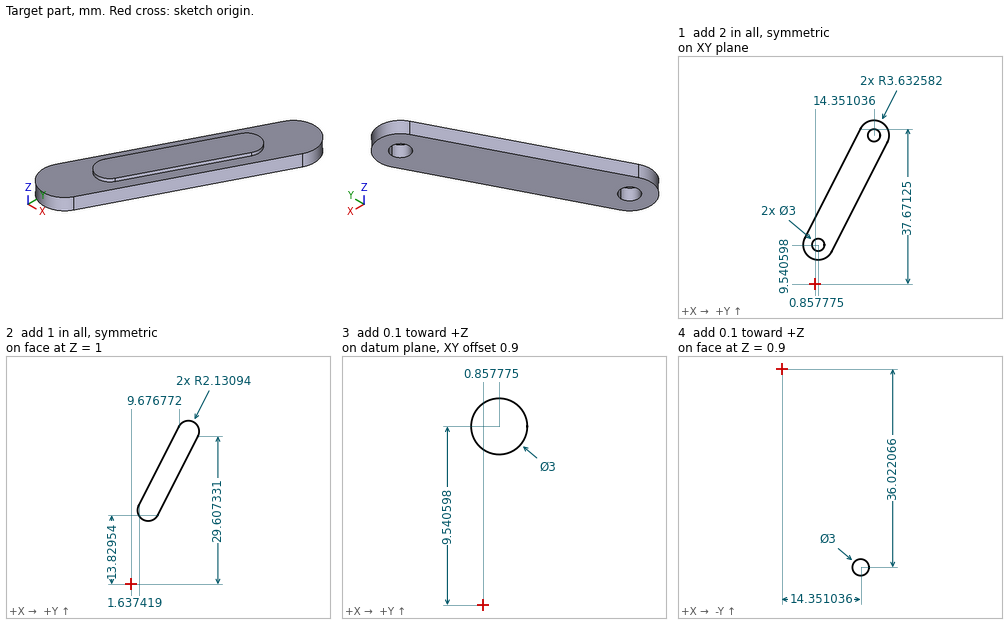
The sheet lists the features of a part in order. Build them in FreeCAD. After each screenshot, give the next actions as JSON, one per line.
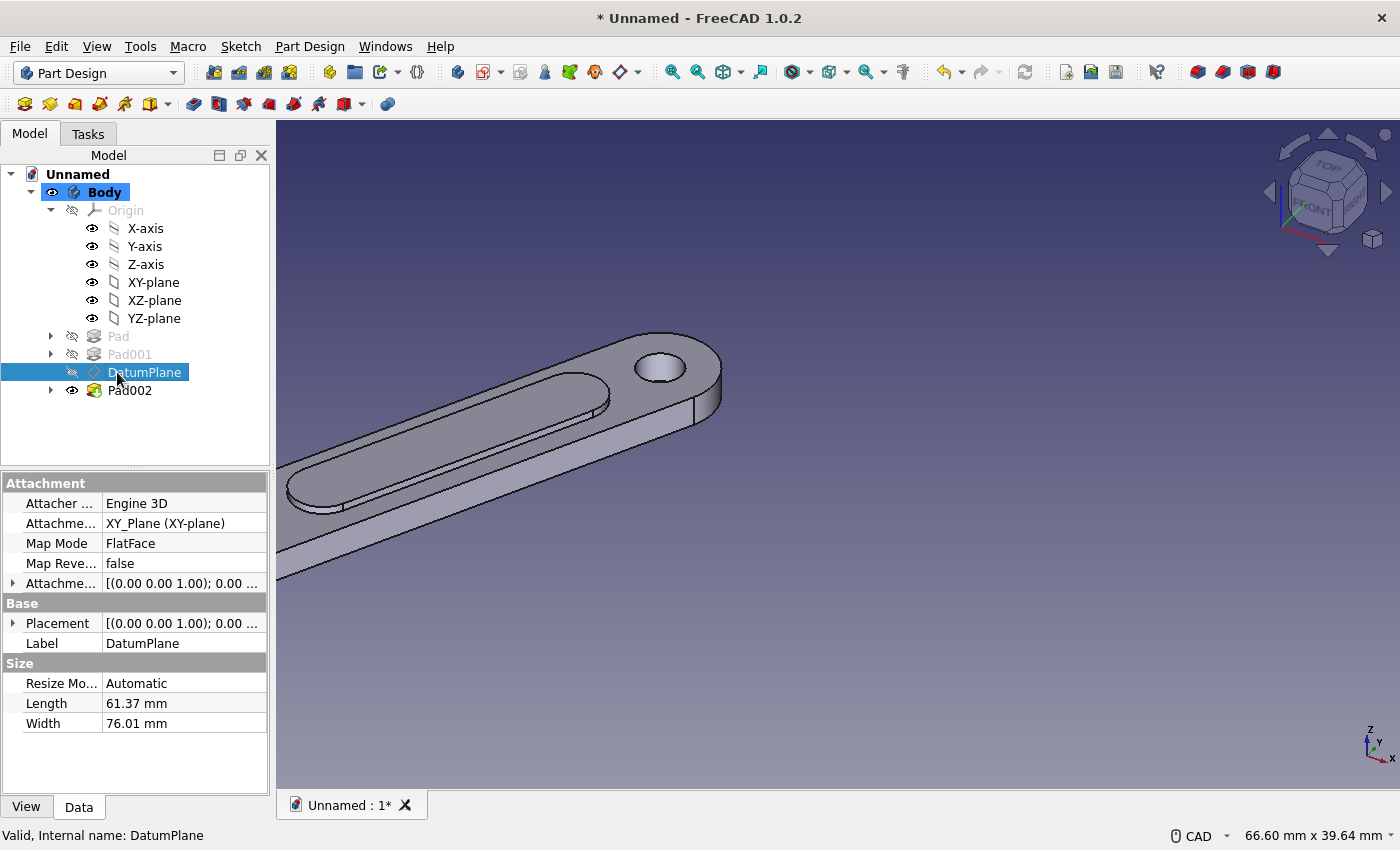
{"action": "key", "text": "v f"}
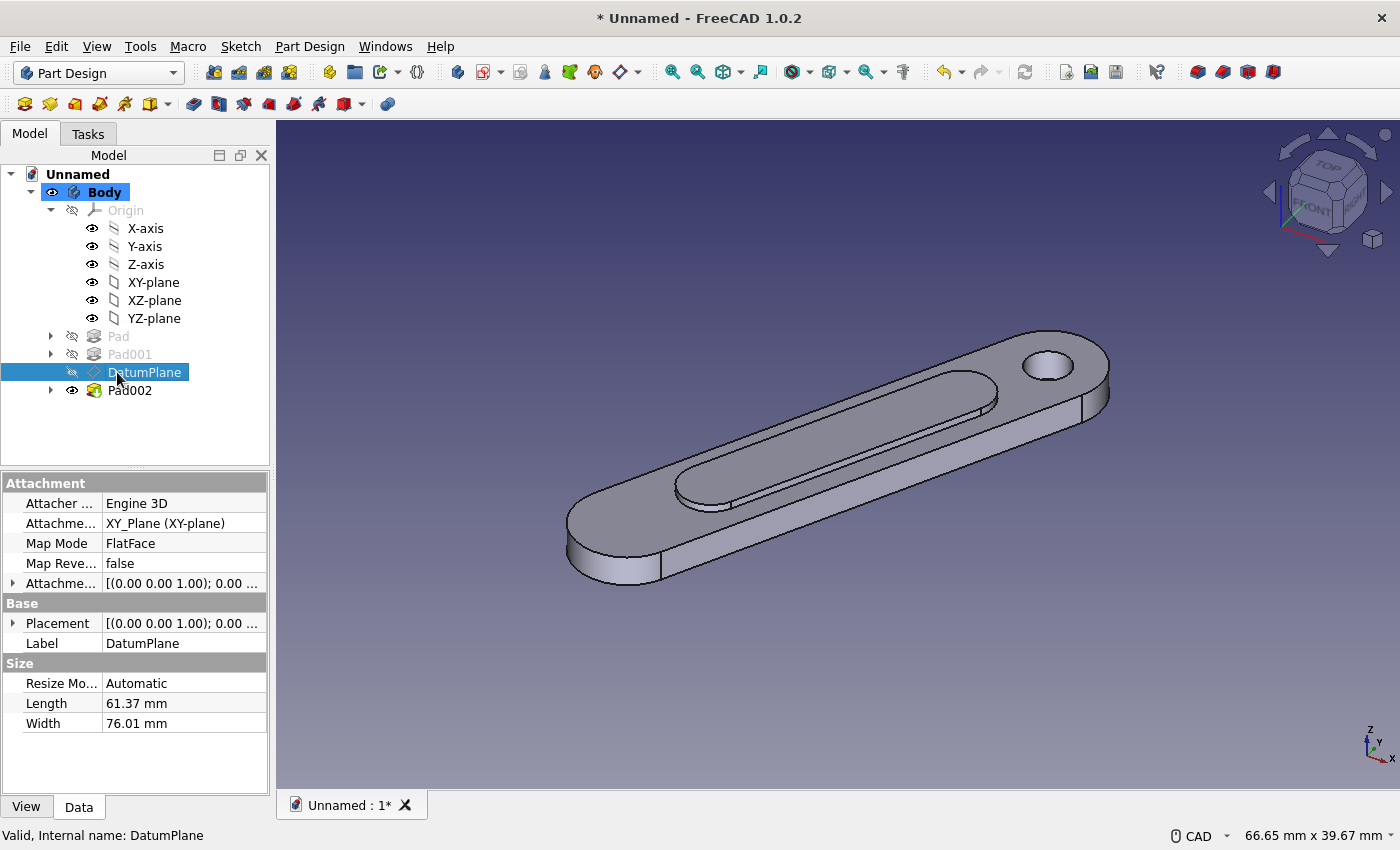
{"action": "key", "text": "5"}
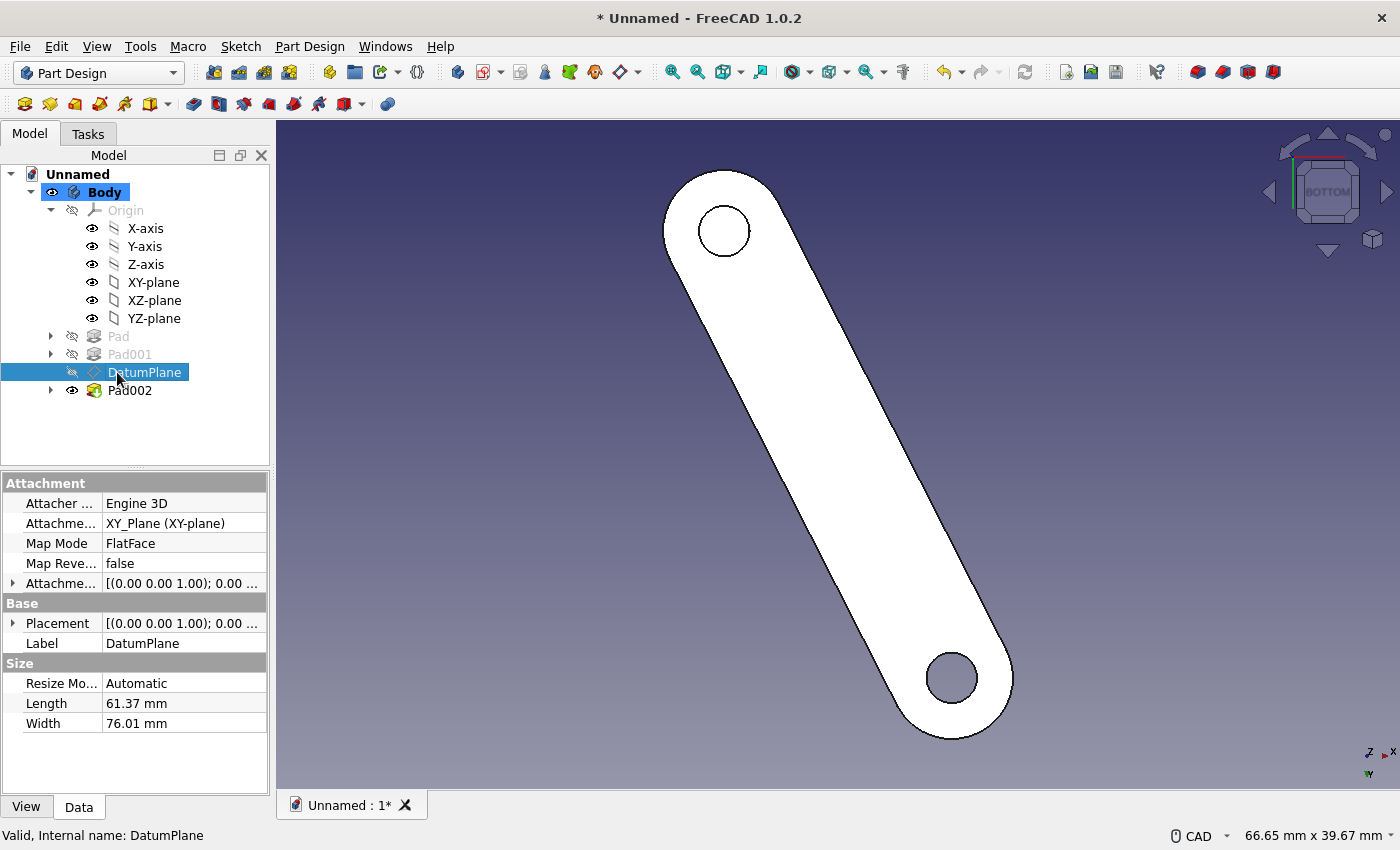
{"action": "left_click", "coordinate": [724, 230]}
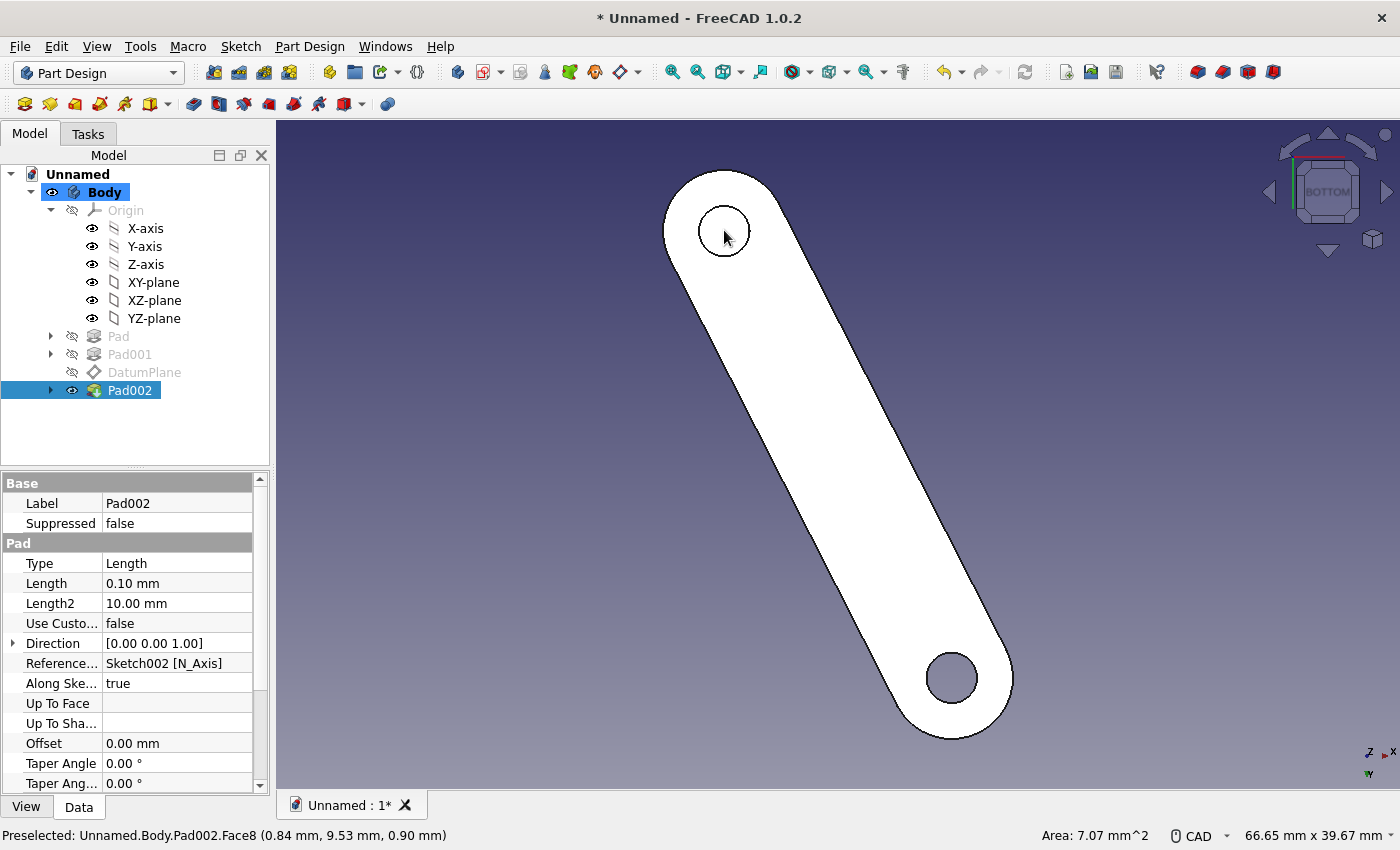
{"action": "left_click", "coordinate": [482, 72]}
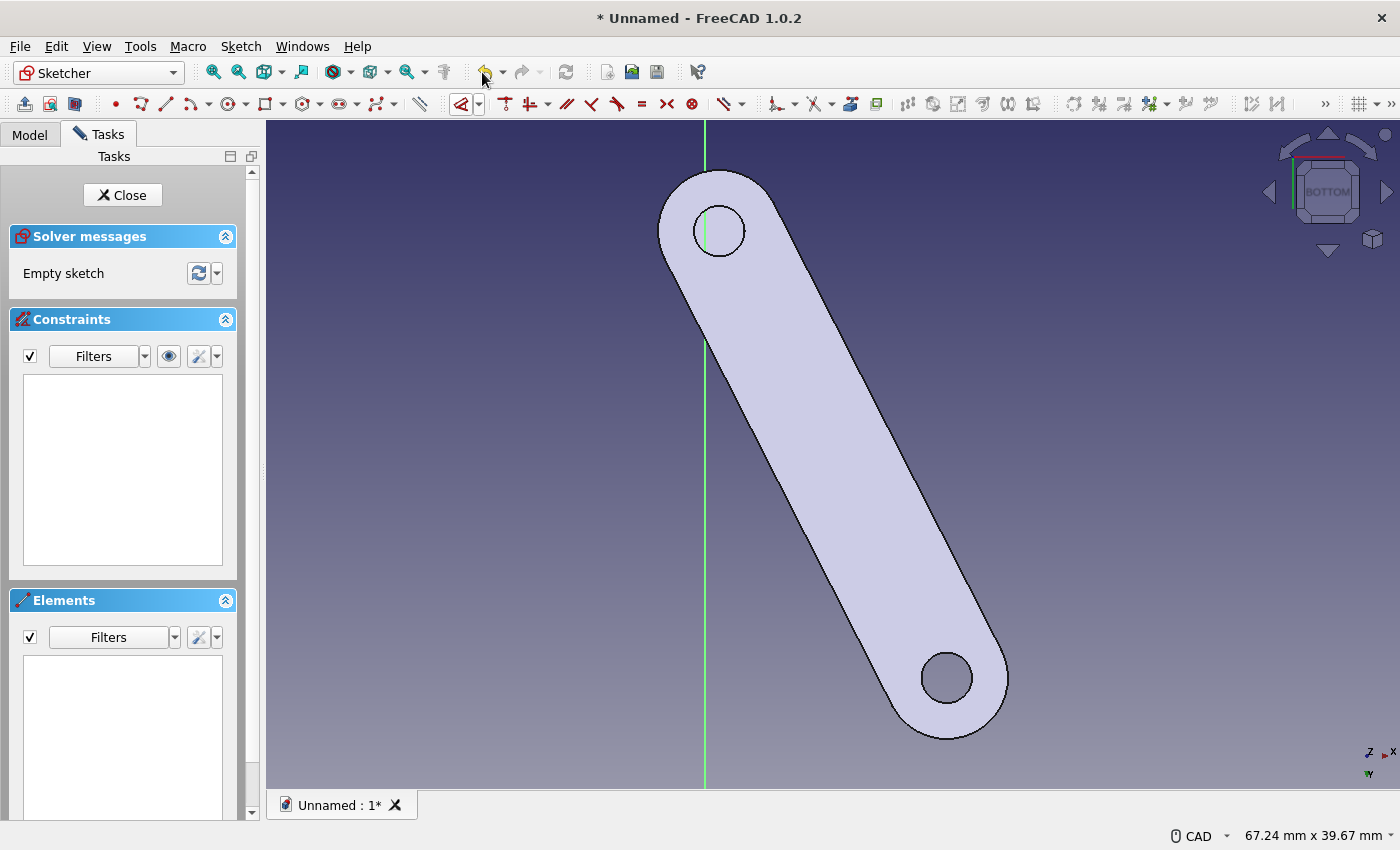
{"action": "scroll", "coordinate": [969, 706], "scroll_direction": "up", "scroll_amount": 11}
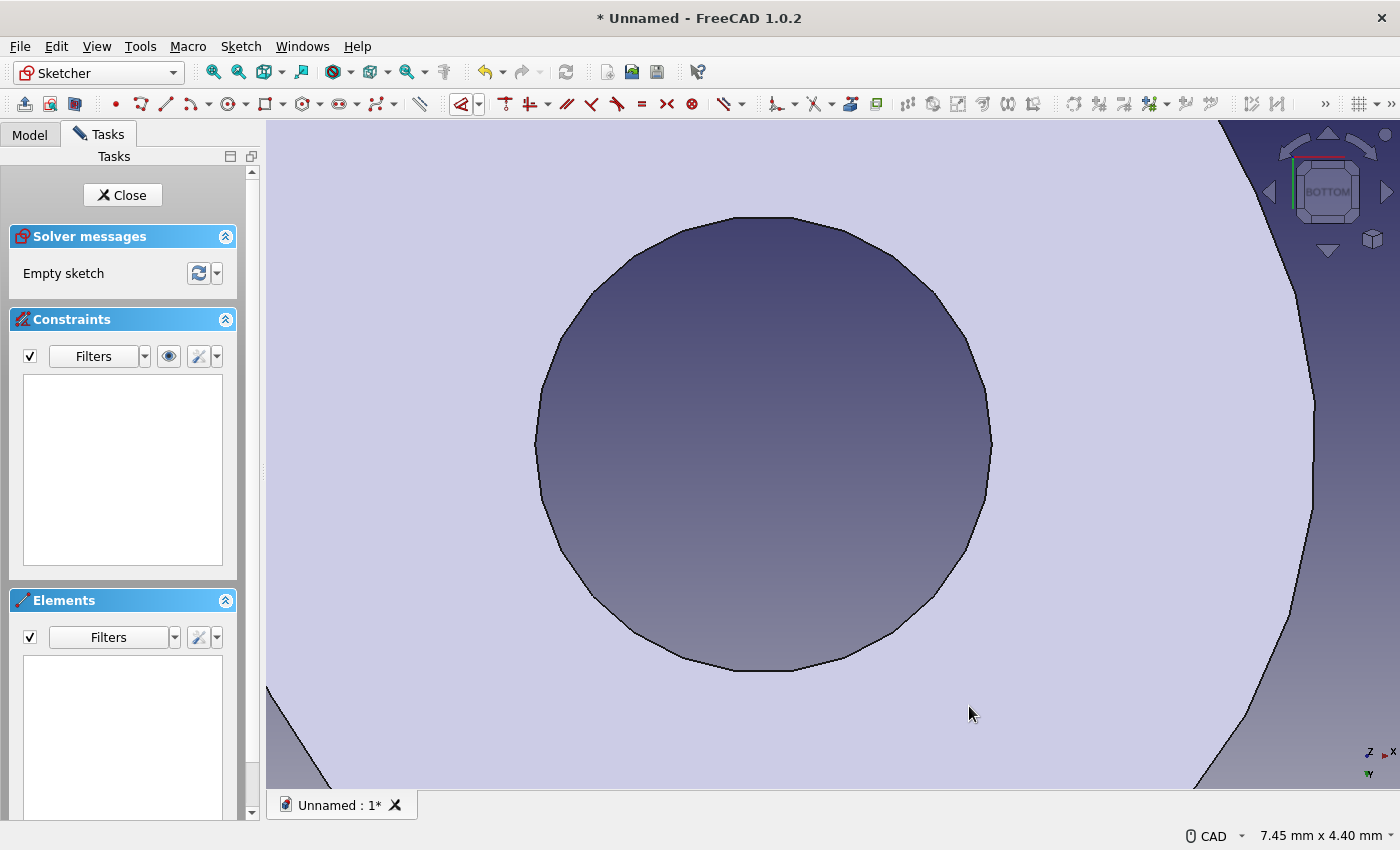
{"action": "key", "text": "g c"}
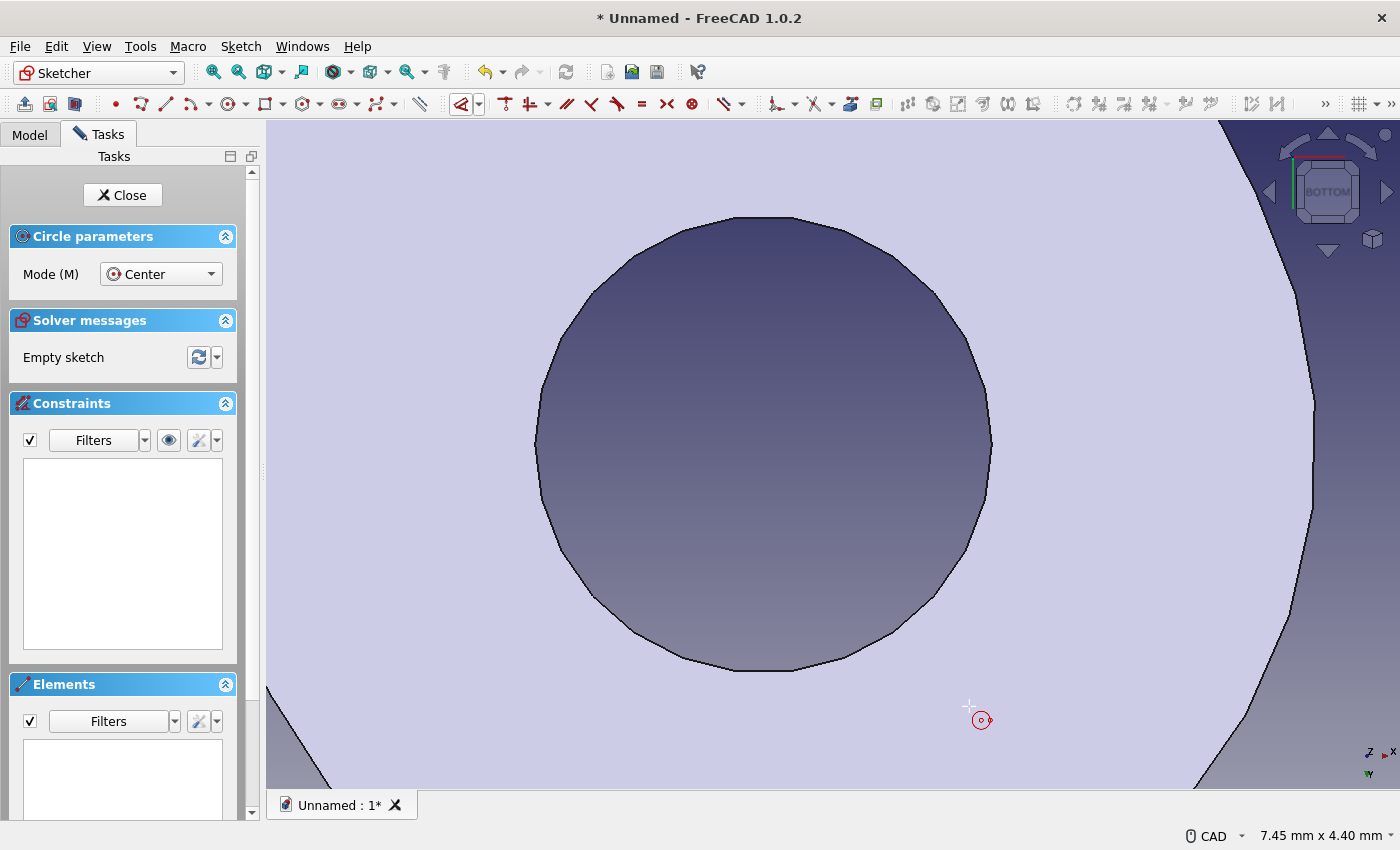
{"action": "left_click", "coordinate": [763, 444]}
{"action": "left_click", "coordinate": [925, 283]}
{"action": "key", "text": "Escape"}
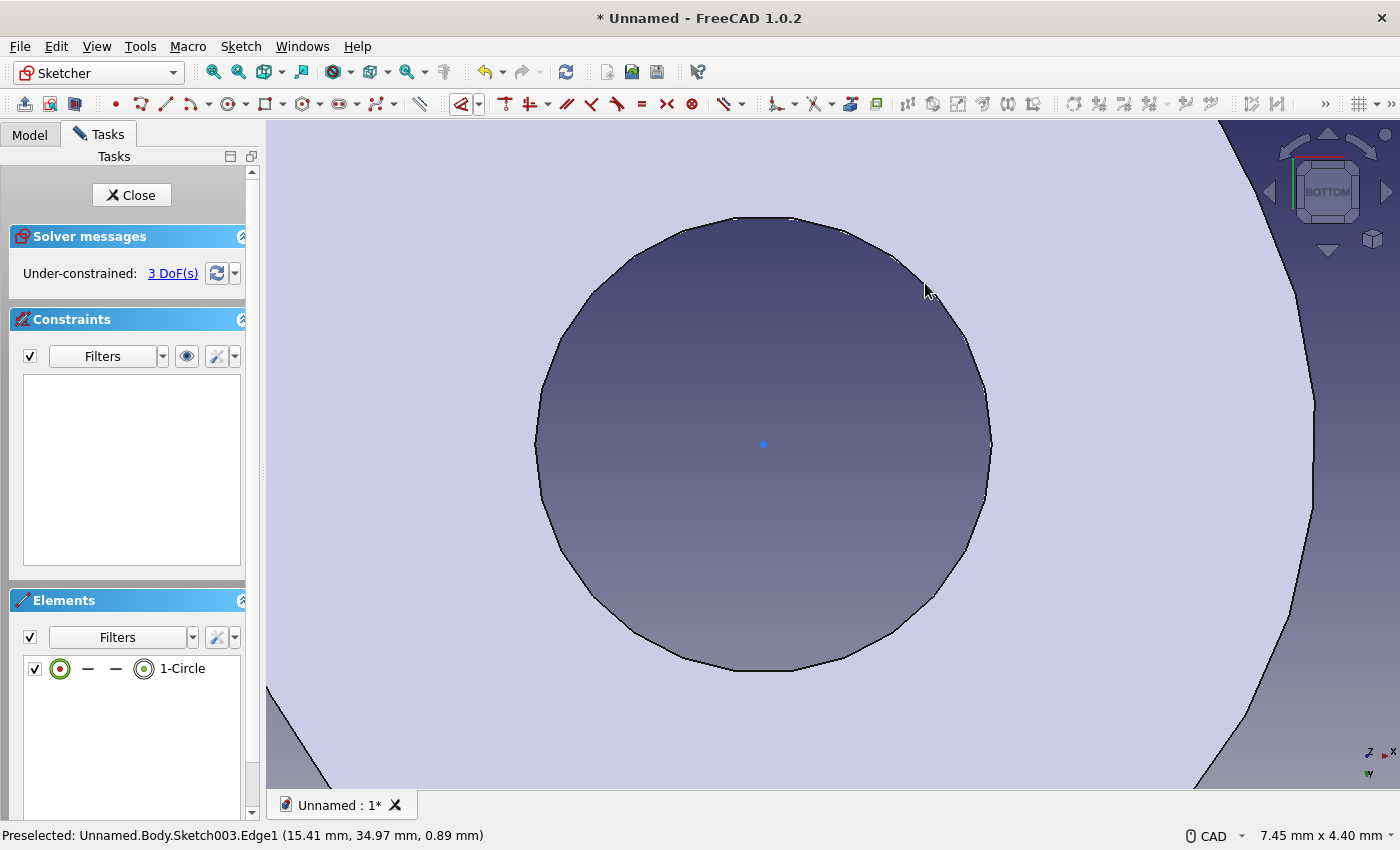
{"action": "left_click", "coordinate": [924, 283]}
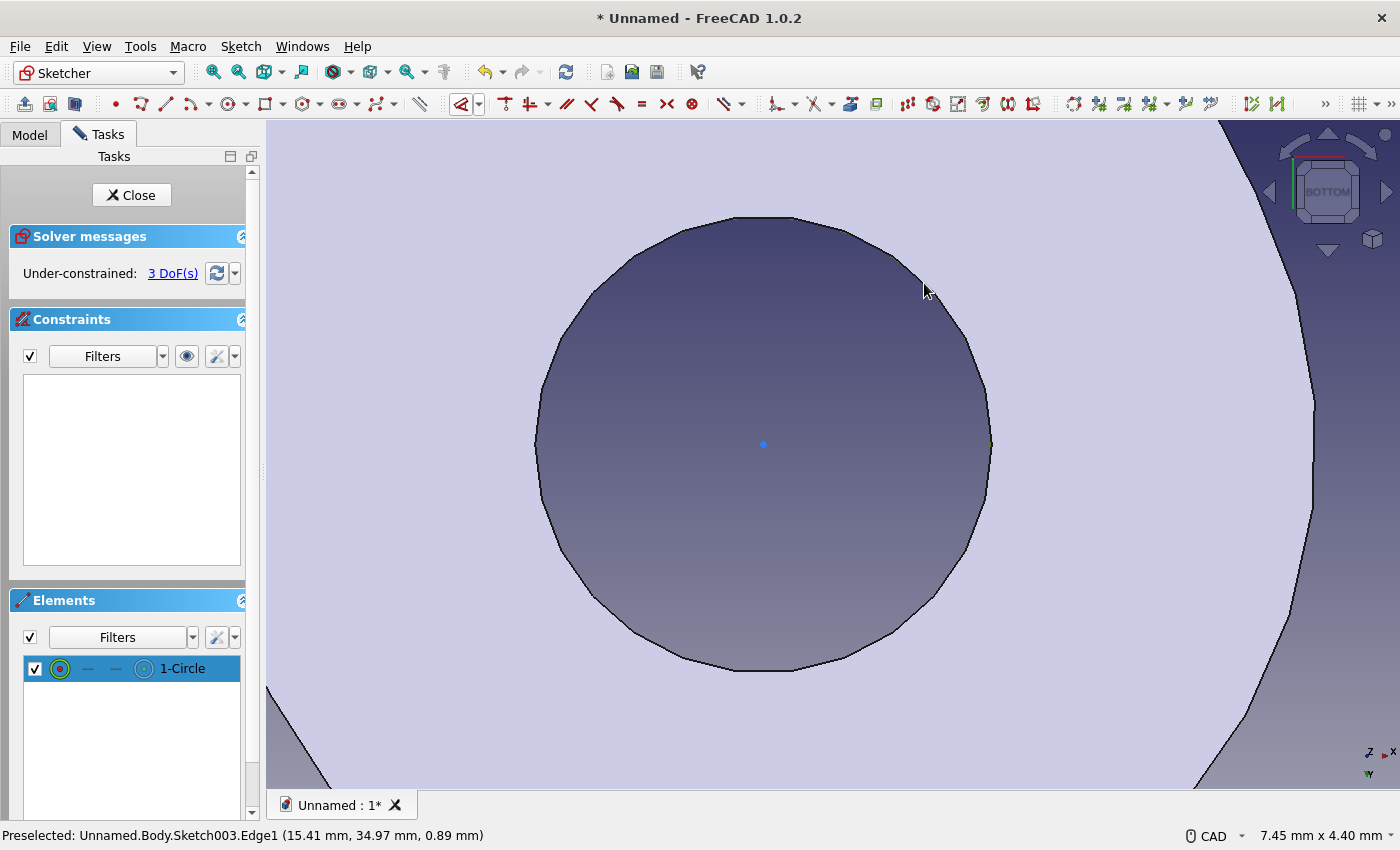
{"action": "key", "text": "k o"}